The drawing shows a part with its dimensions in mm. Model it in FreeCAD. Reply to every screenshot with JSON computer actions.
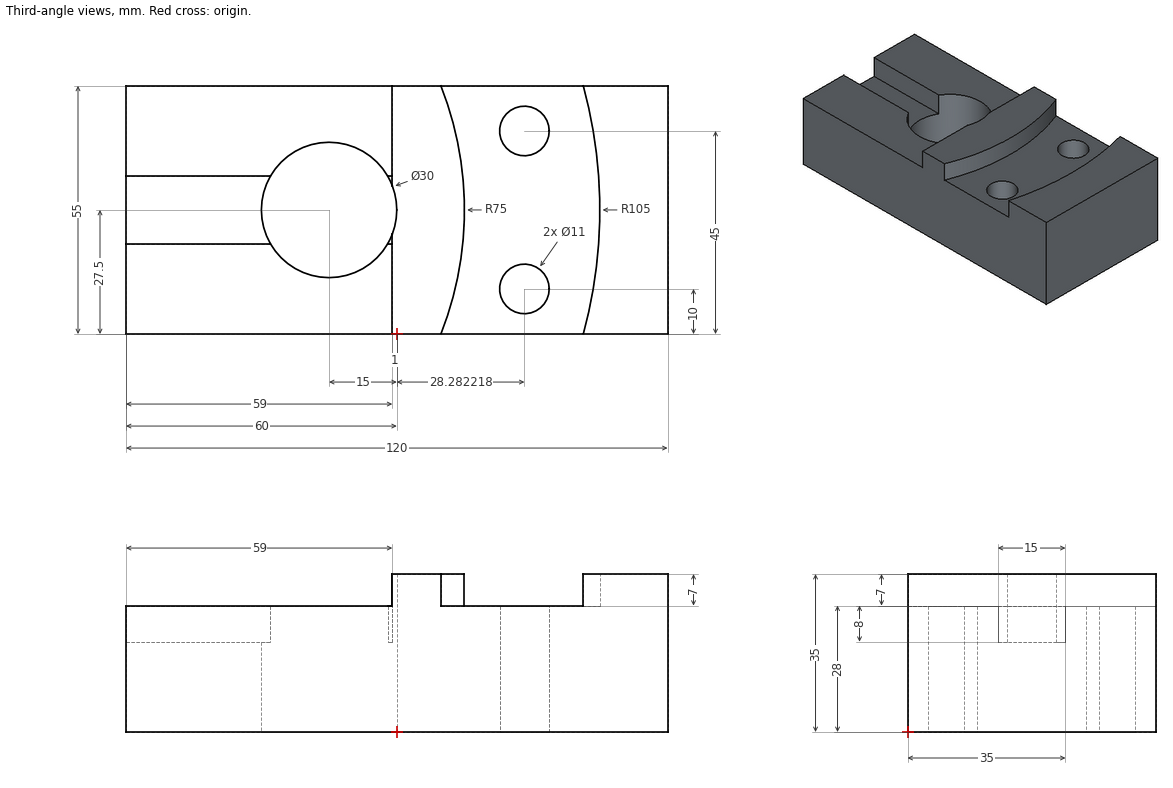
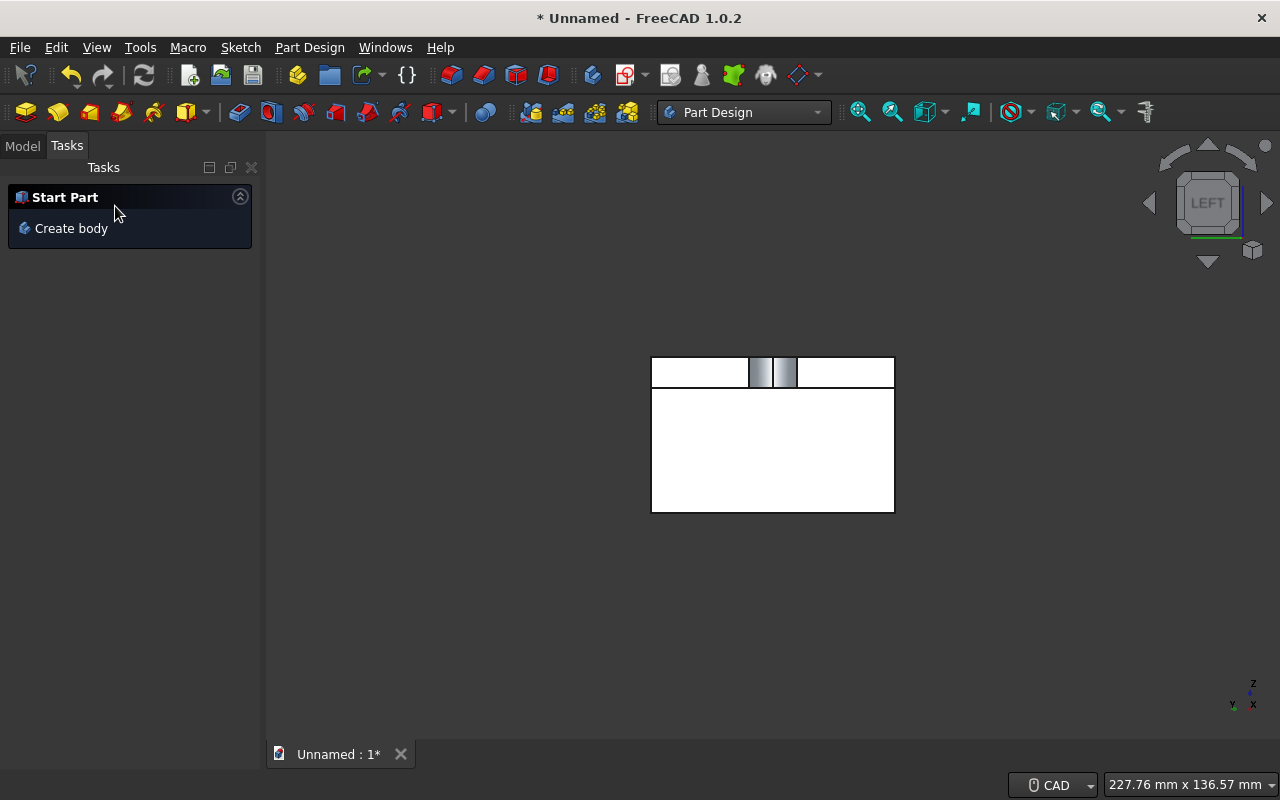
{"action": "key", "text": "v f"}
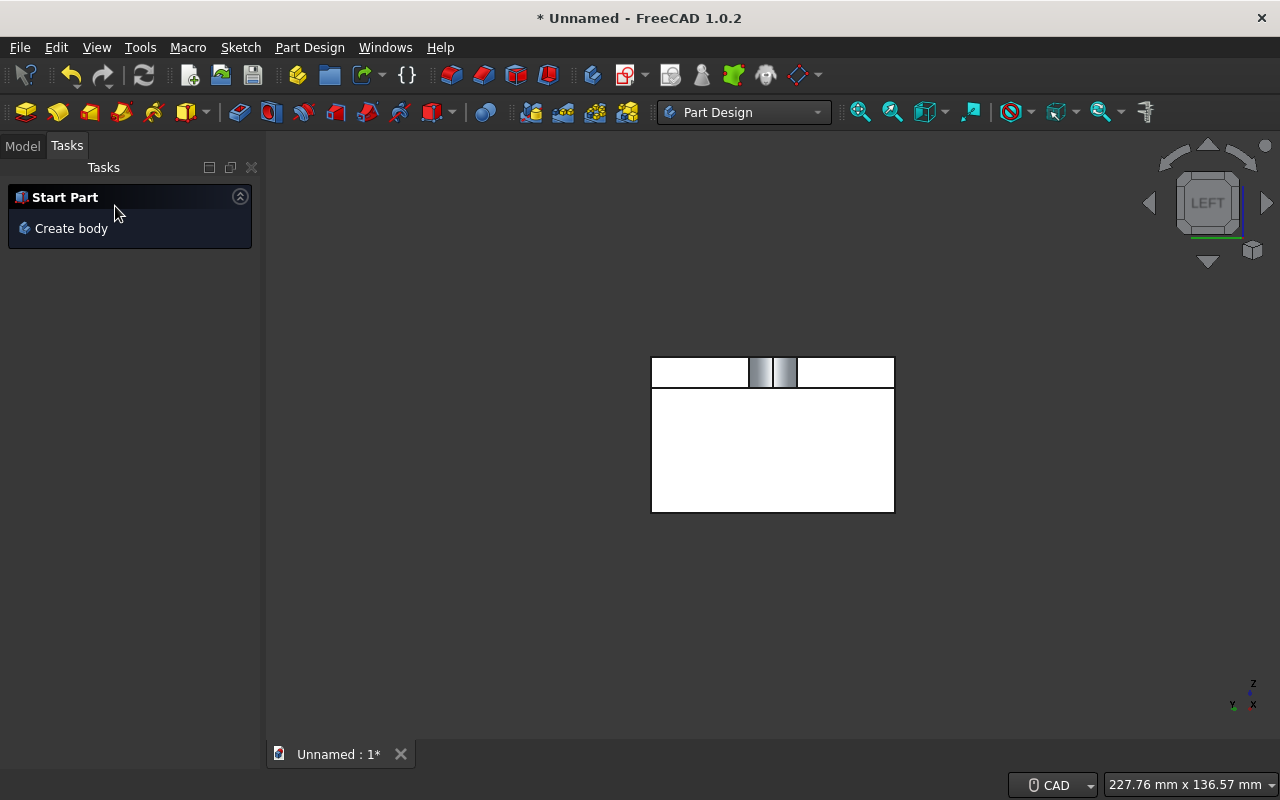
{"action": "left_click", "coordinate": [738, 450]}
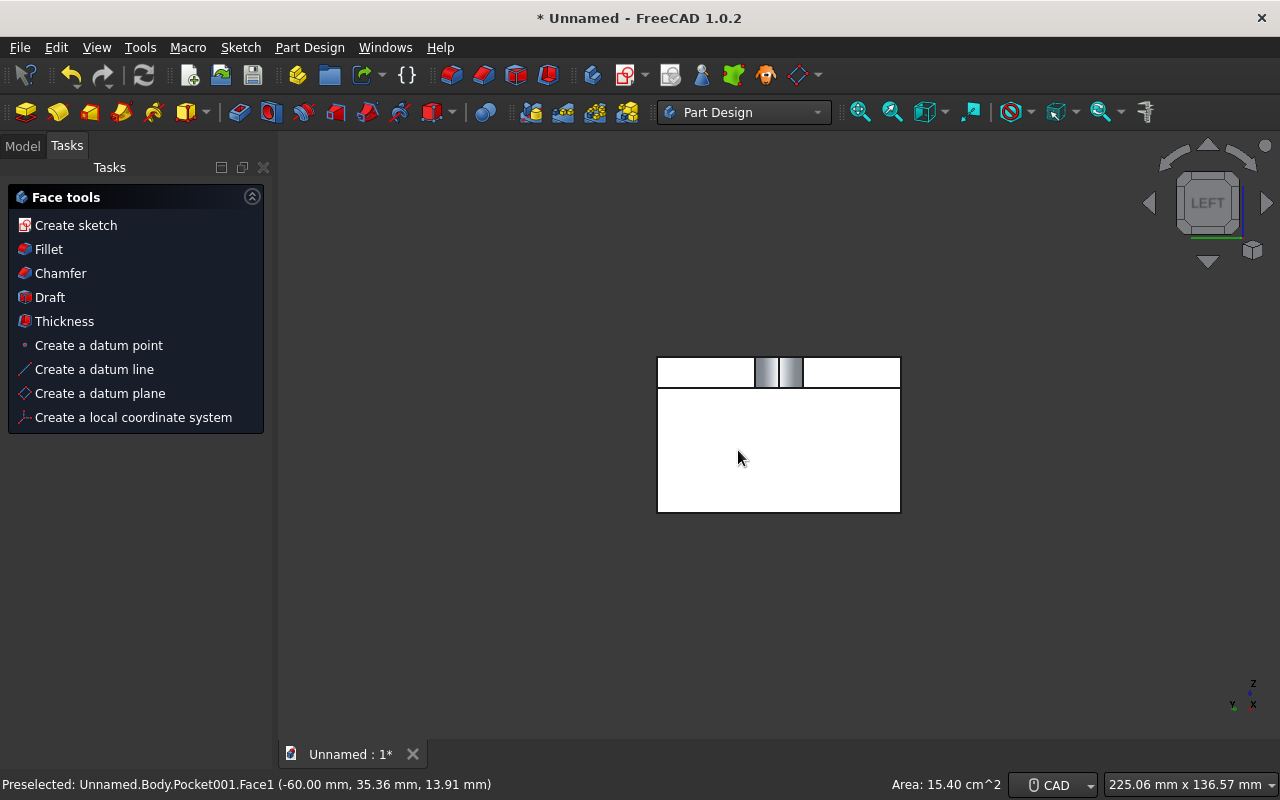
{"action": "left_click", "coordinate": [626, 76]}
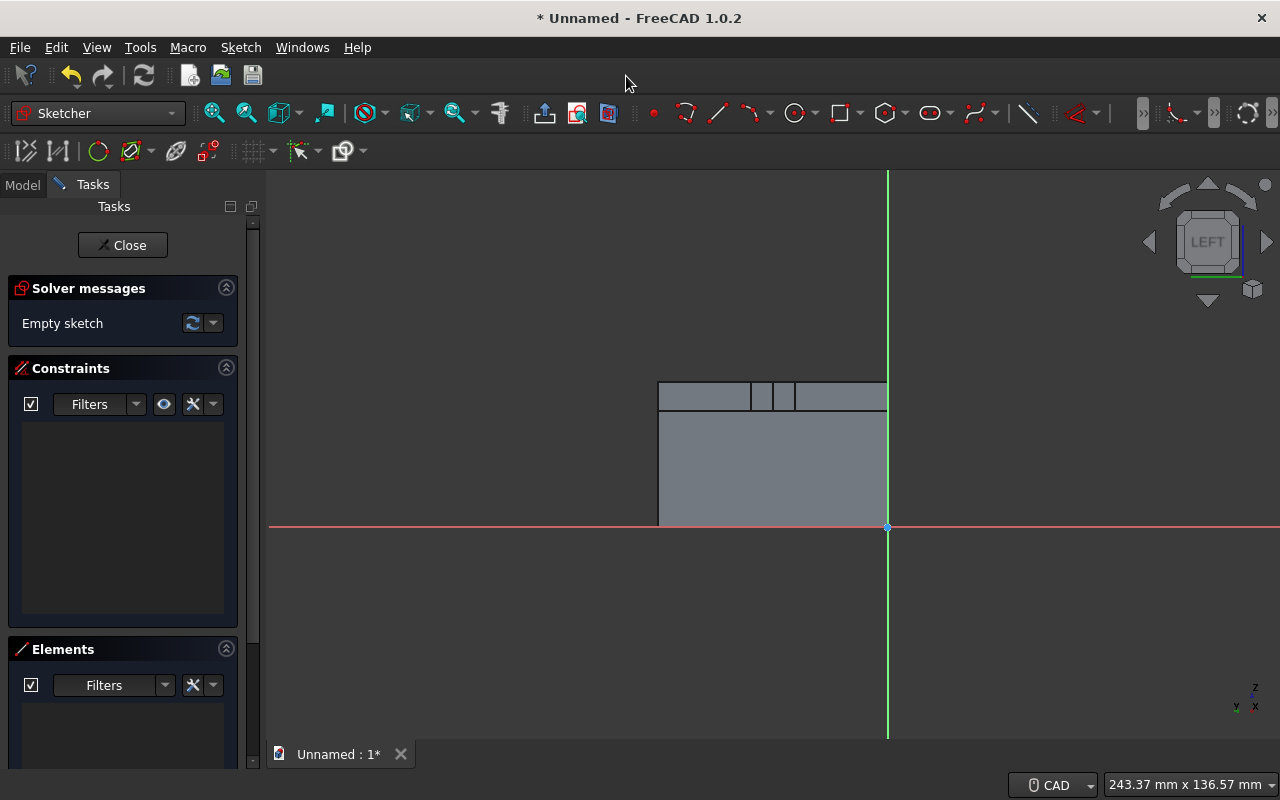
{"action": "scroll", "coordinate": [862, 475], "scroll_direction": "up", "scroll_amount": 6}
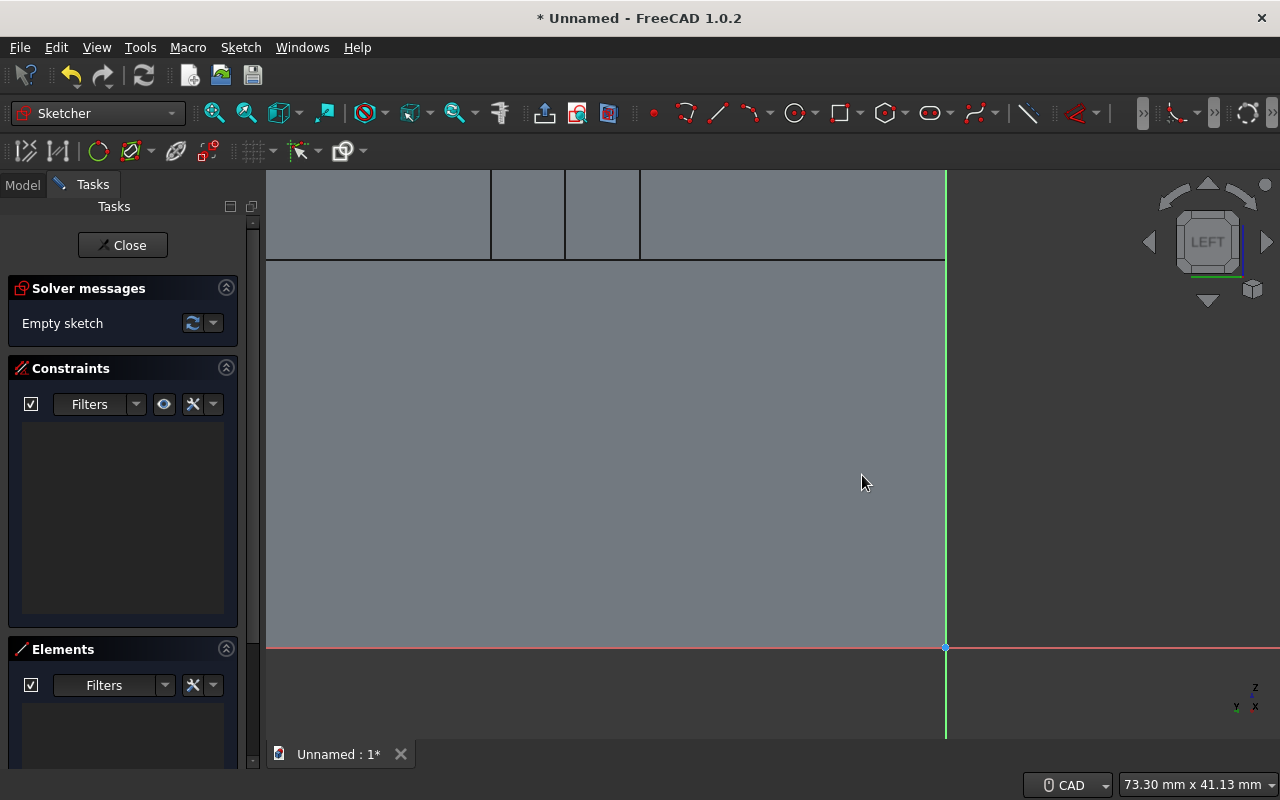
{"action": "key", "text": "g r"}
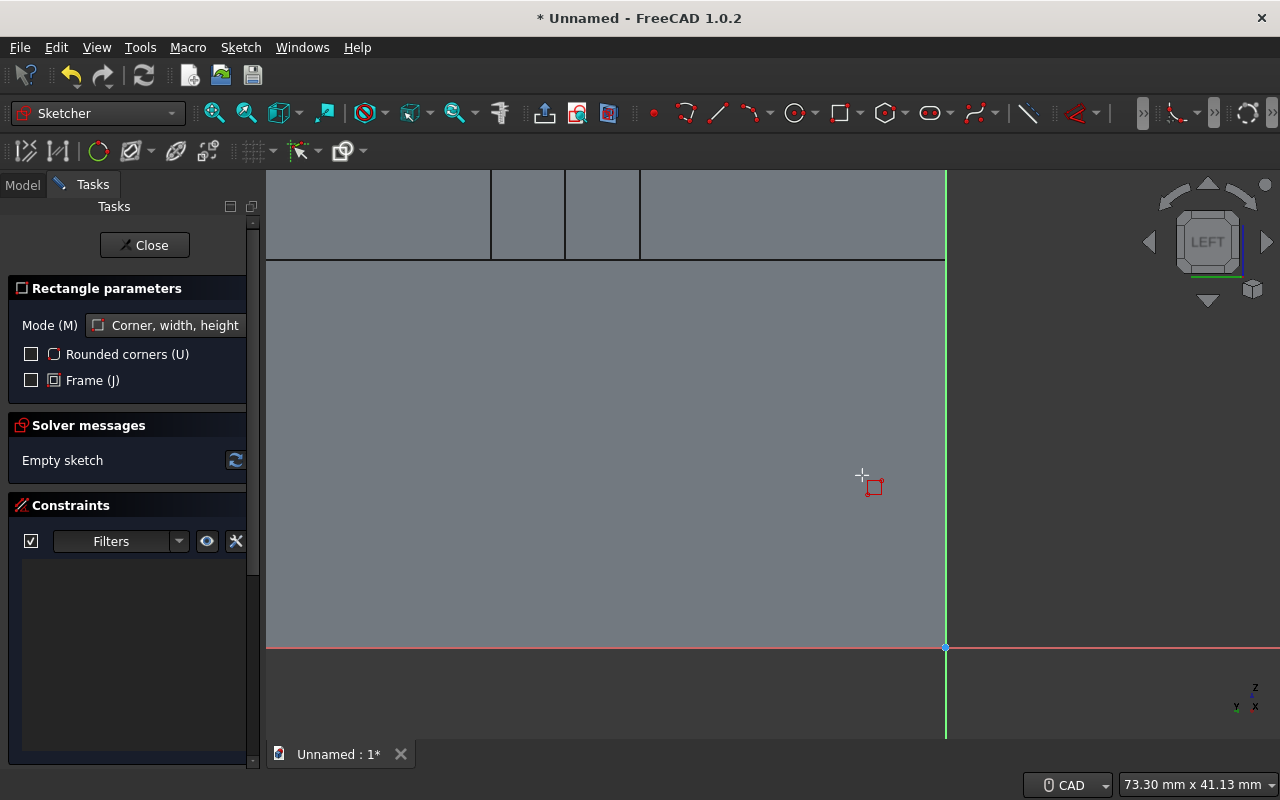
{"action": "left_click", "coordinate": [461, 260]}
{"action": "mouse_move", "coordinate": [669, 371]}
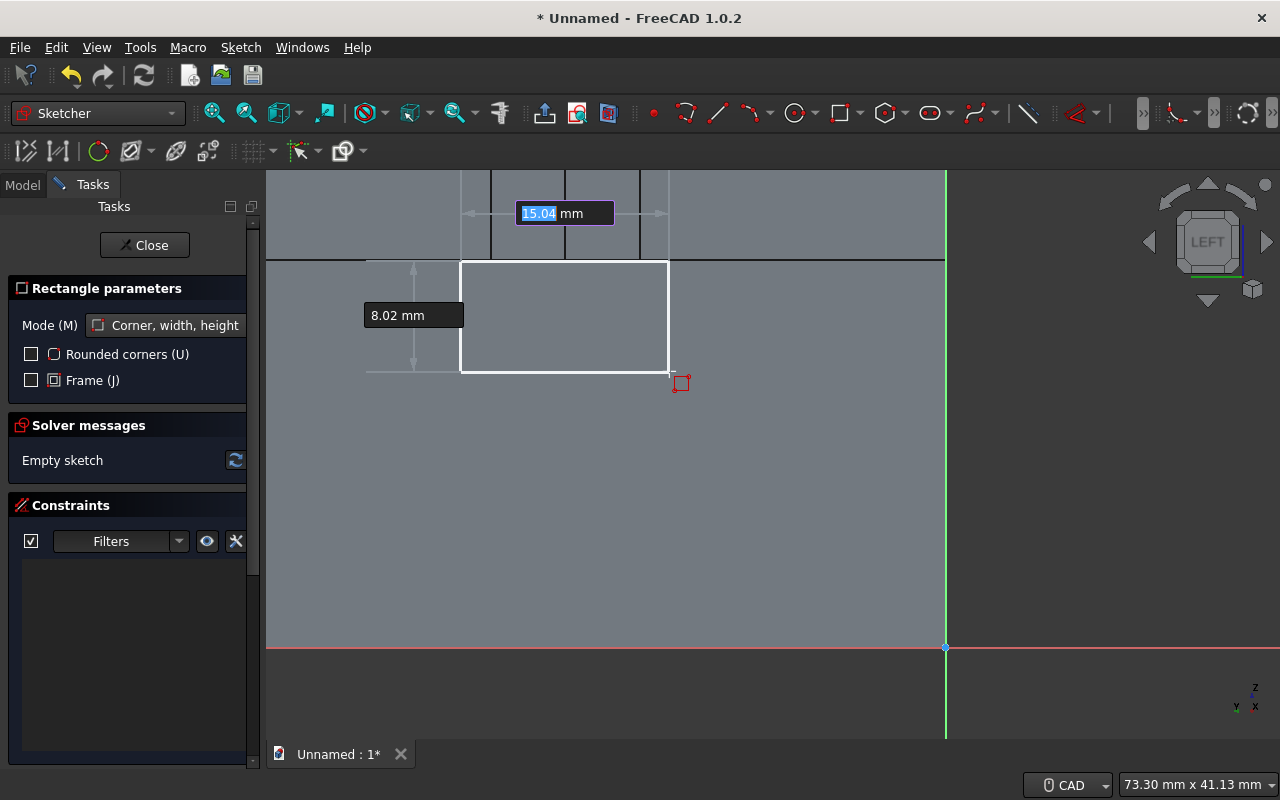
{"action": "type", "text": "15"}
{"action": "key", "text": "Tab"}
{"action": "type", "text": "8"}
{"action": "key", "text": "Return"}
{"action": "key", "text": "Escape"}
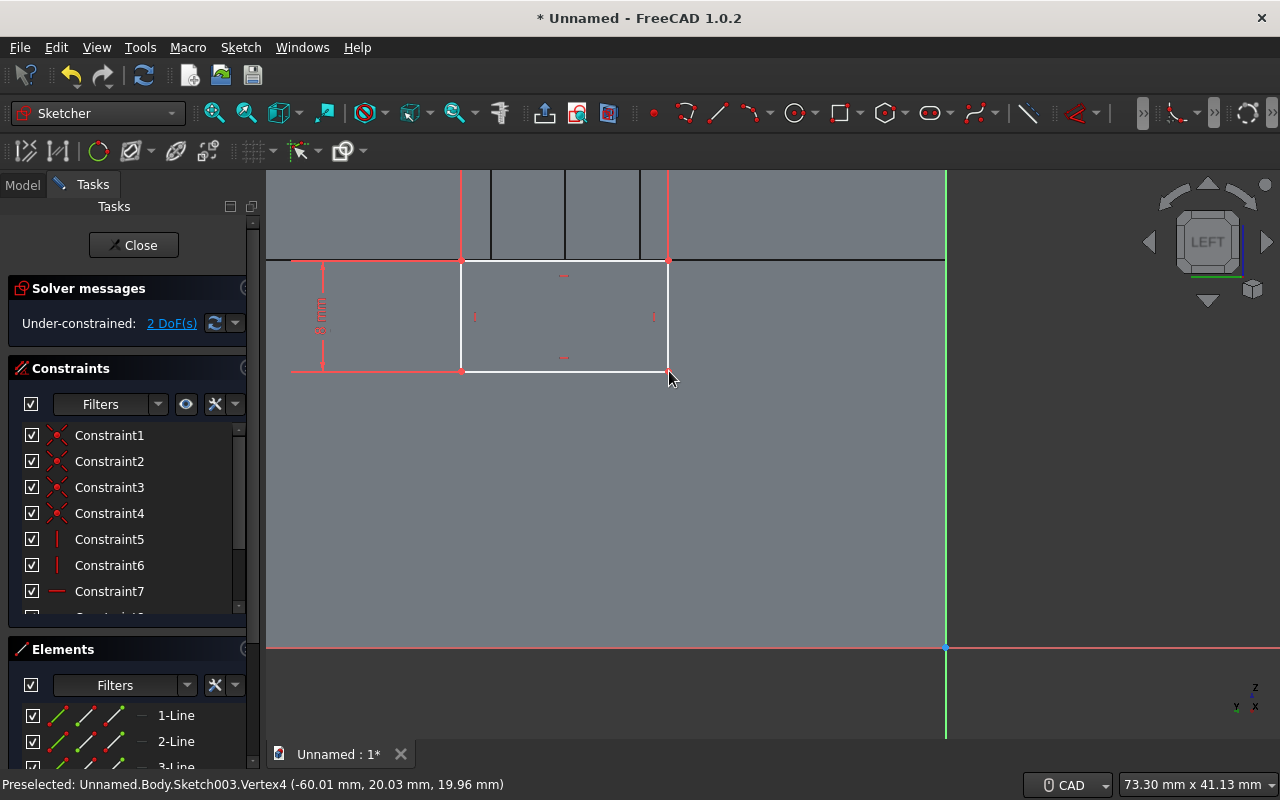
{"action": "key", "text": "d"}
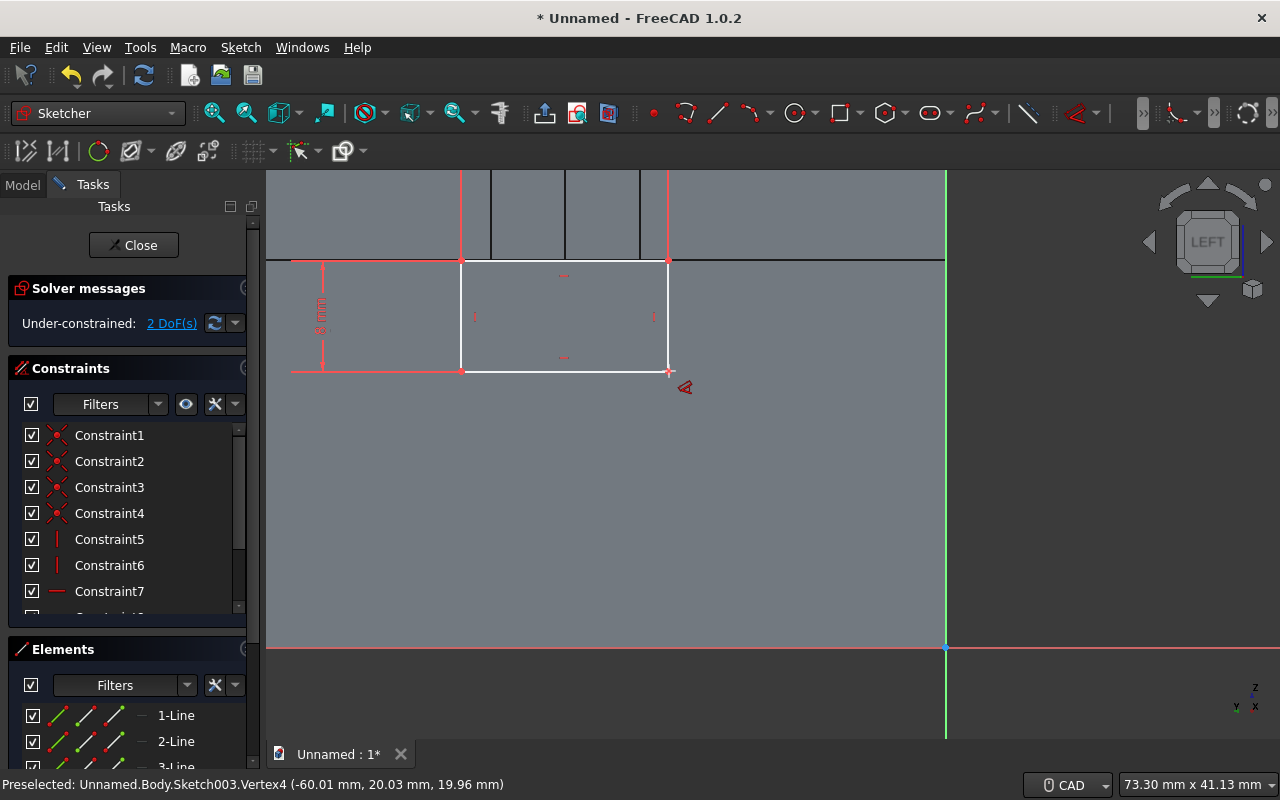
{"action": "left_click", "coordinate": [461, 261]}
{"action": "left_click", "coordinate": [703, 682]}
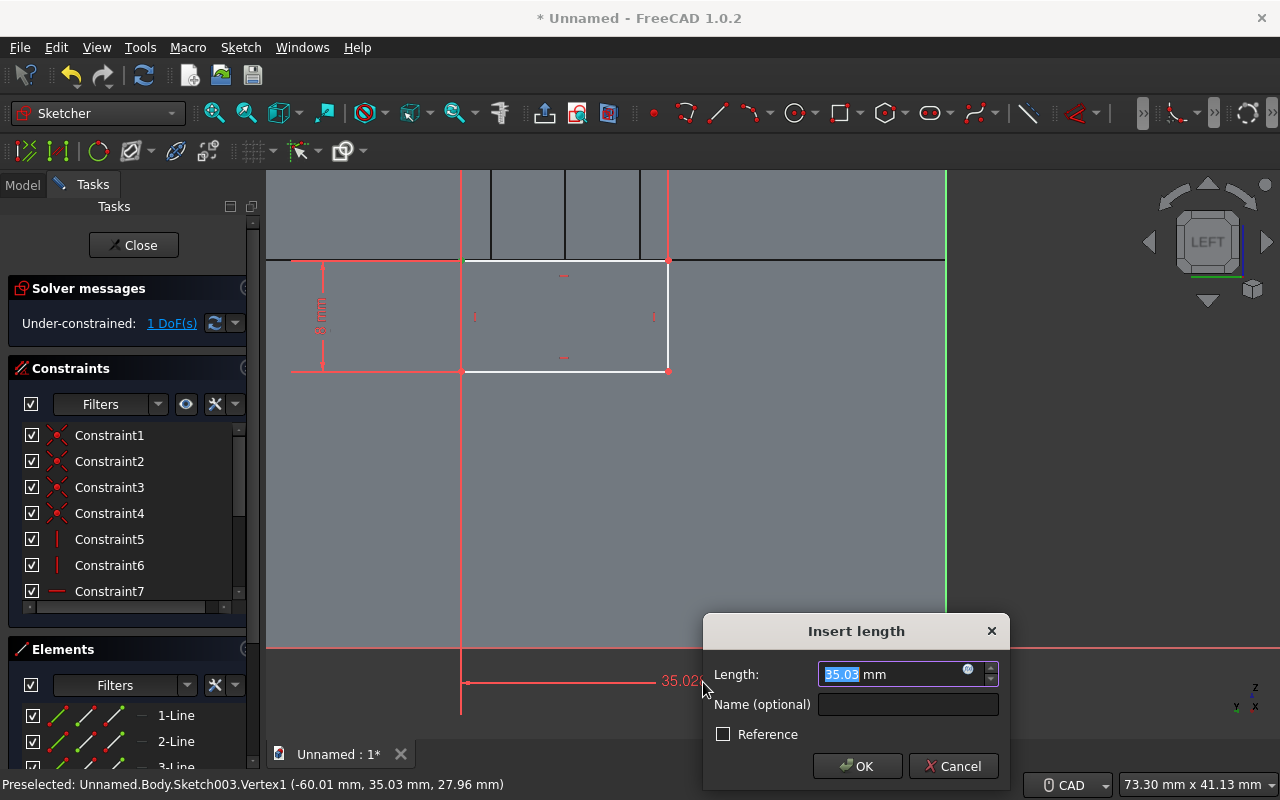
{"action": "type", "text": "35"}
{"action": "key", "text": "Return"}